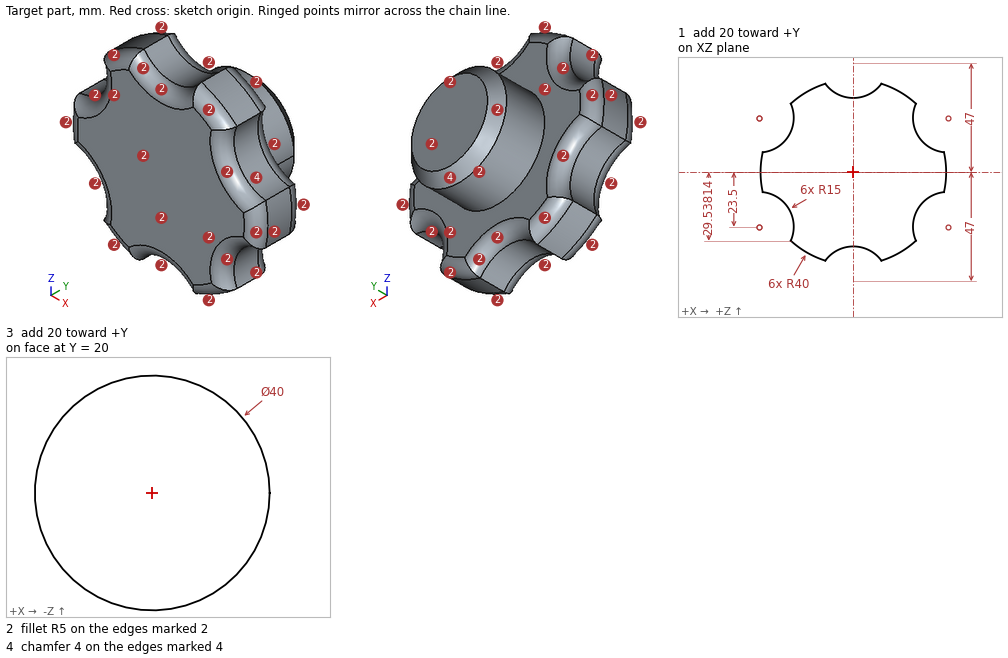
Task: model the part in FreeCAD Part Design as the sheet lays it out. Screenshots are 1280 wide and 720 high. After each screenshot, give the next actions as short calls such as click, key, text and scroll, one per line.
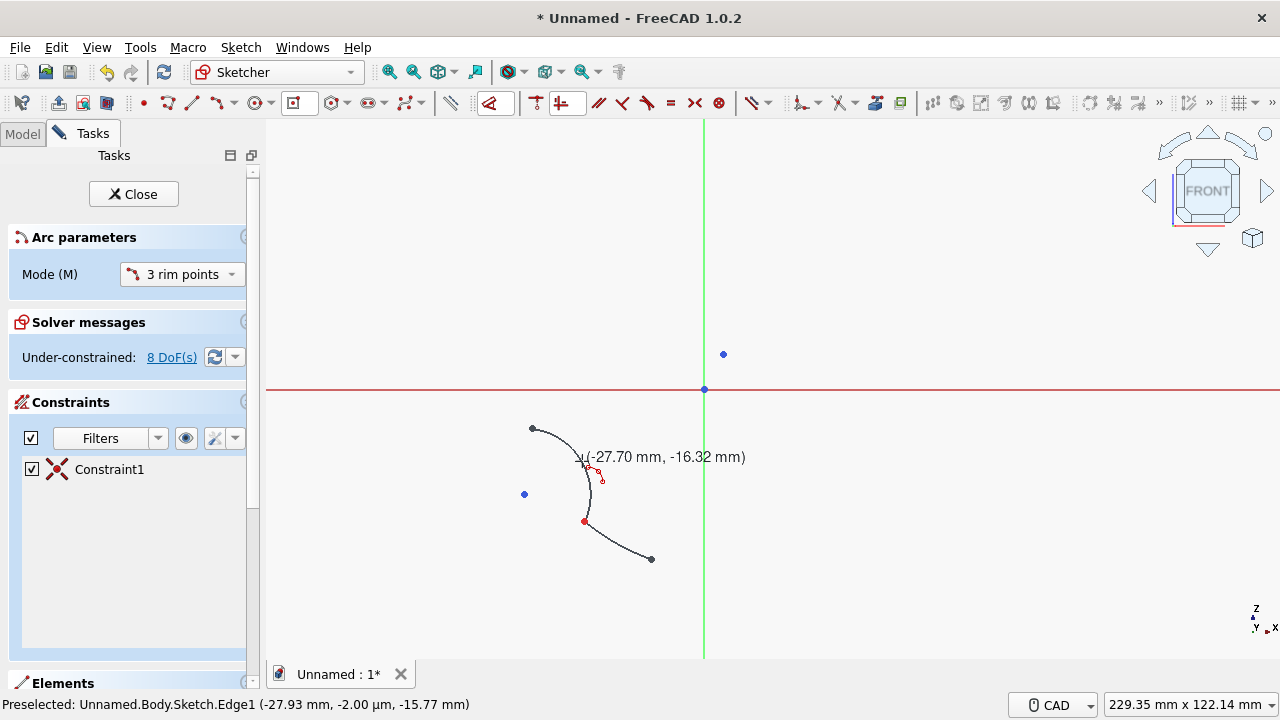
click(532, 429)
click(532, 352)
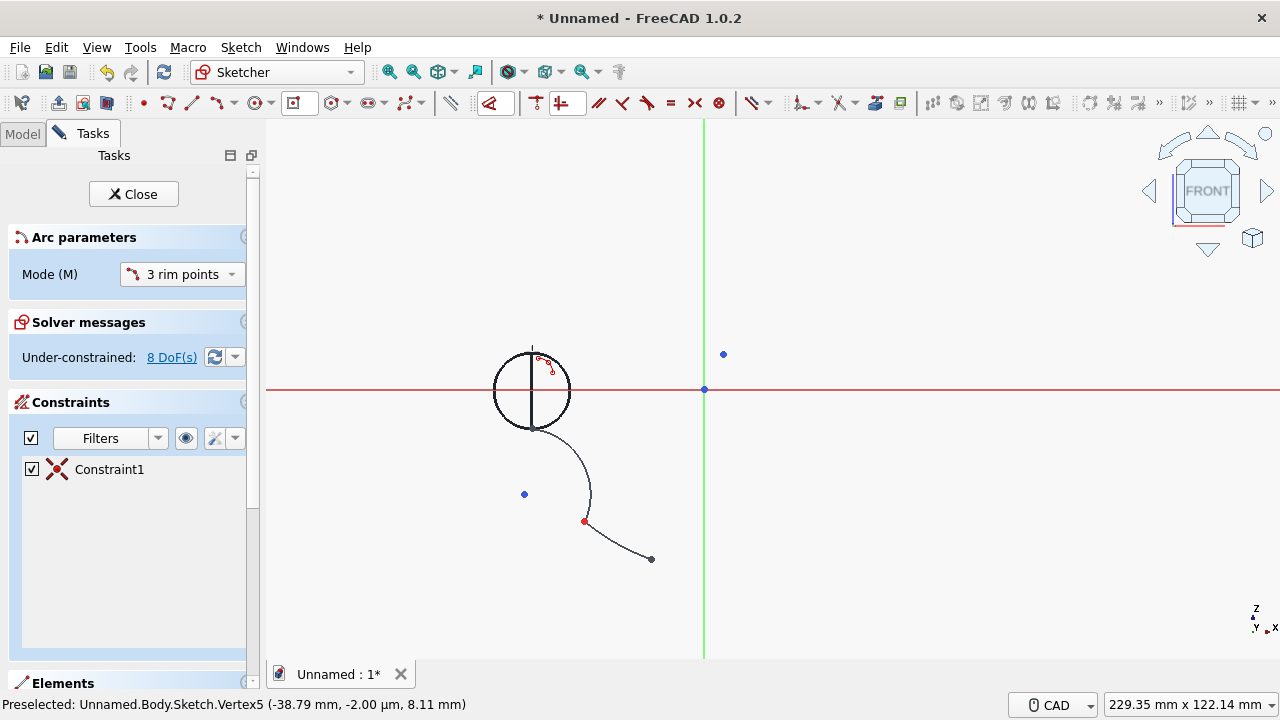
scroll(528, 382, up, 7)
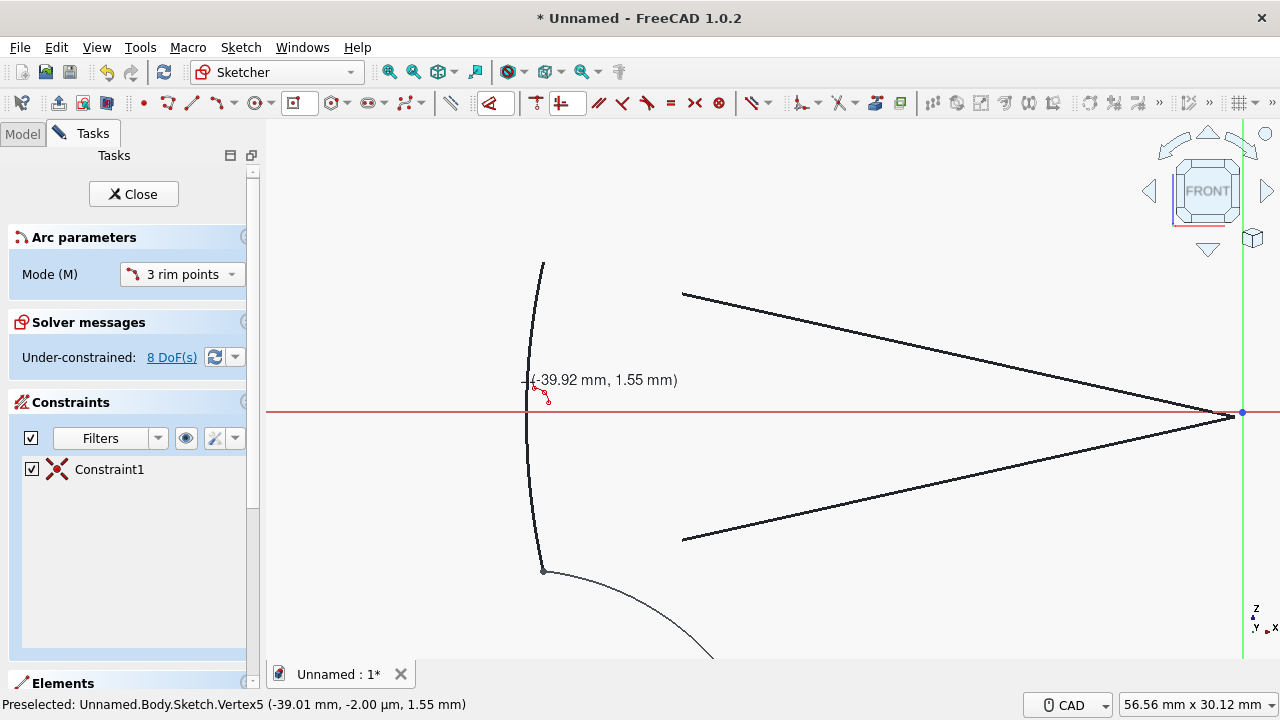
click(526, 381)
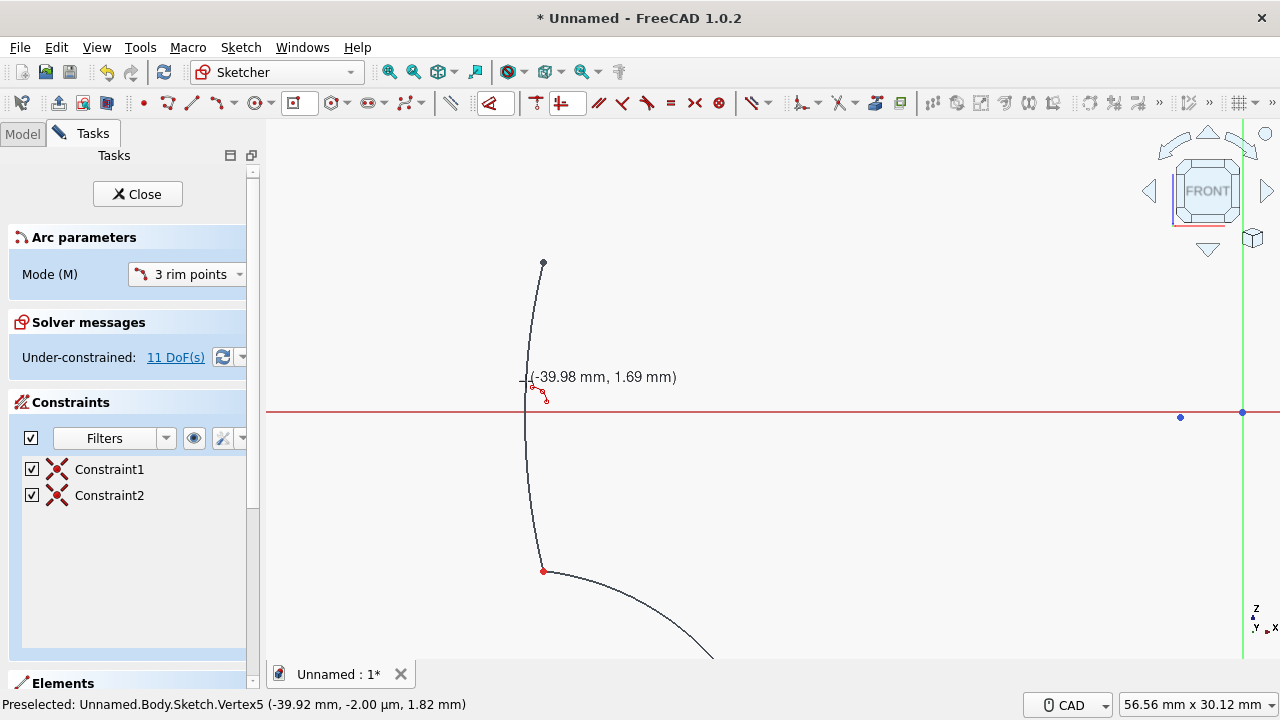
click(543, 263)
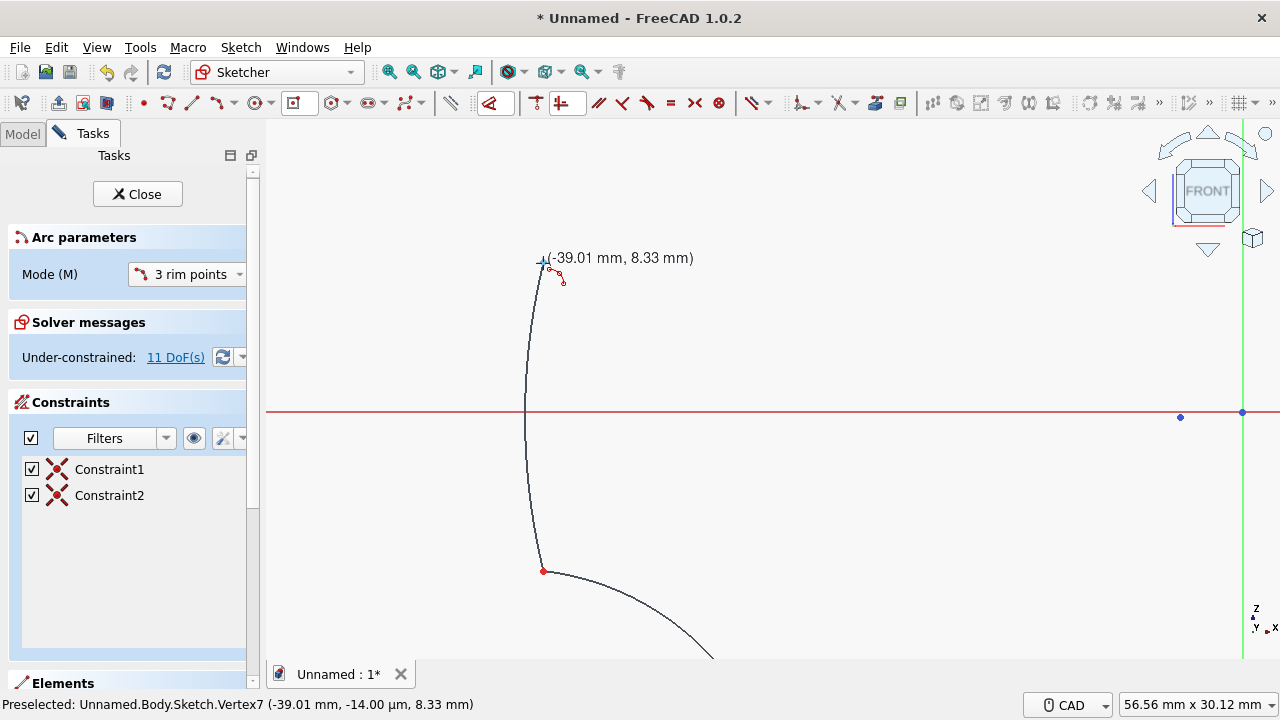
scroll(528, 381, down, 7)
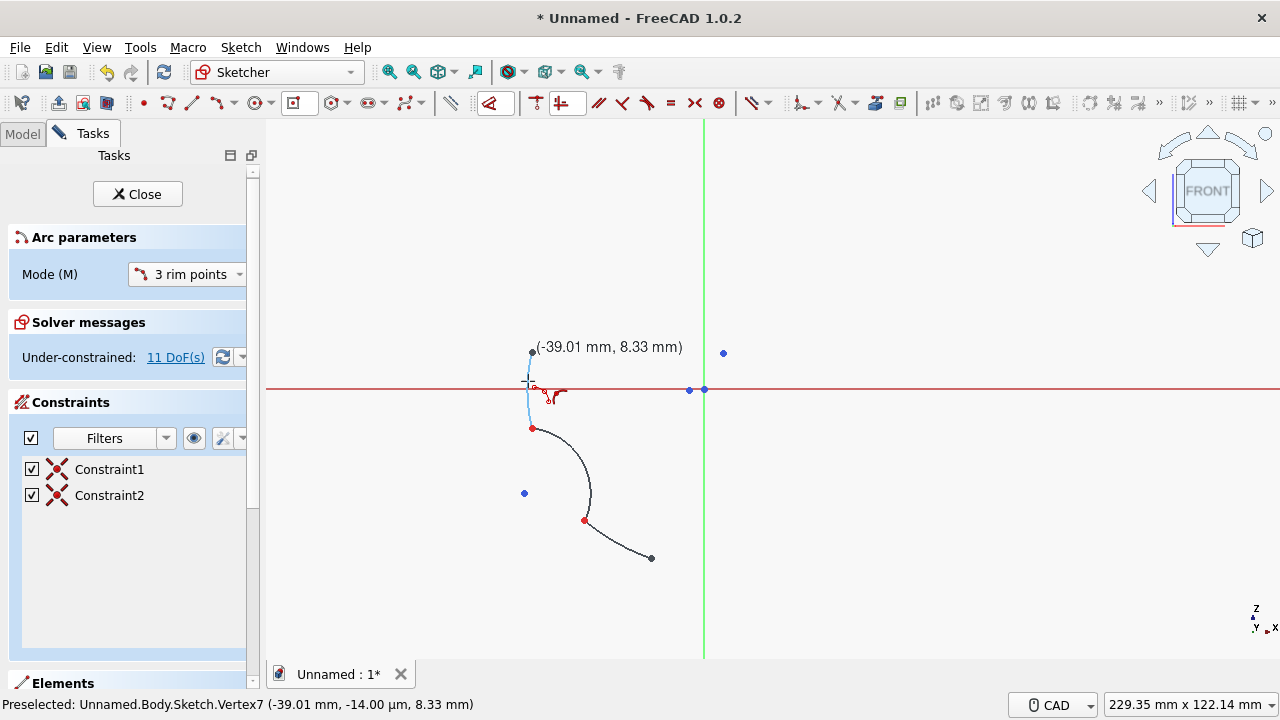
click(585, 258)
click(582, 318)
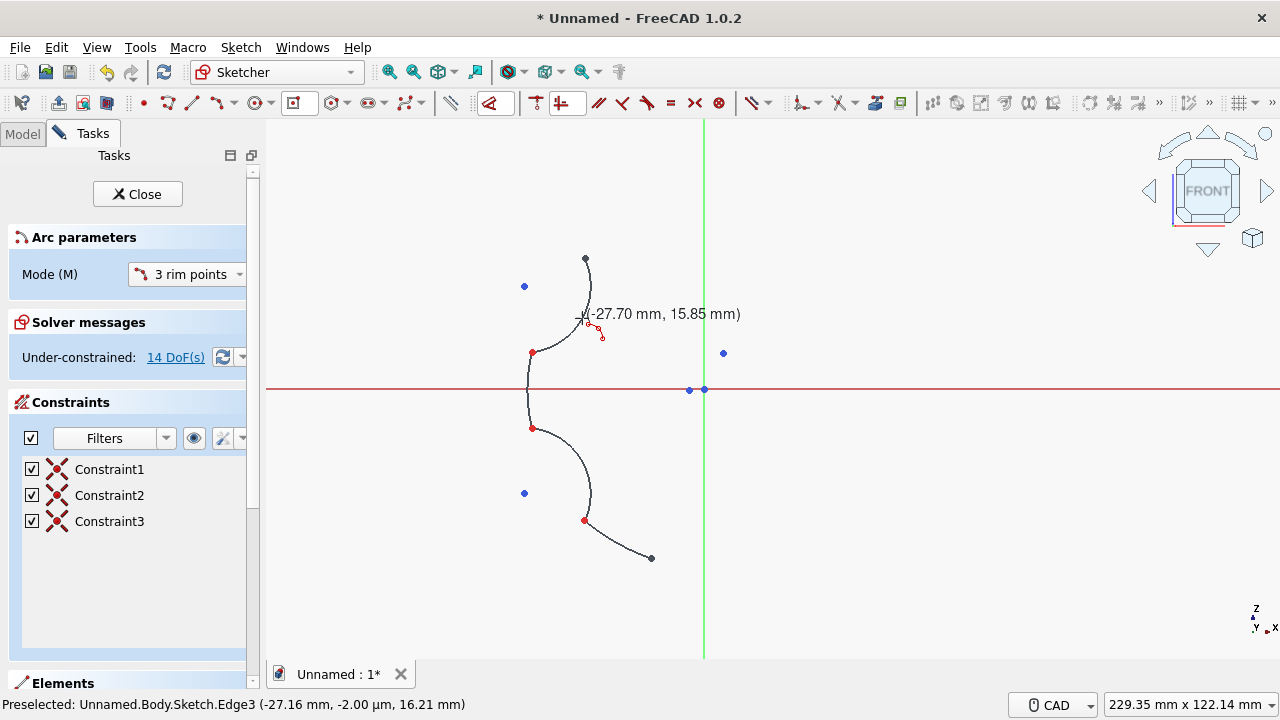
click(585, 259)
click(651, 221)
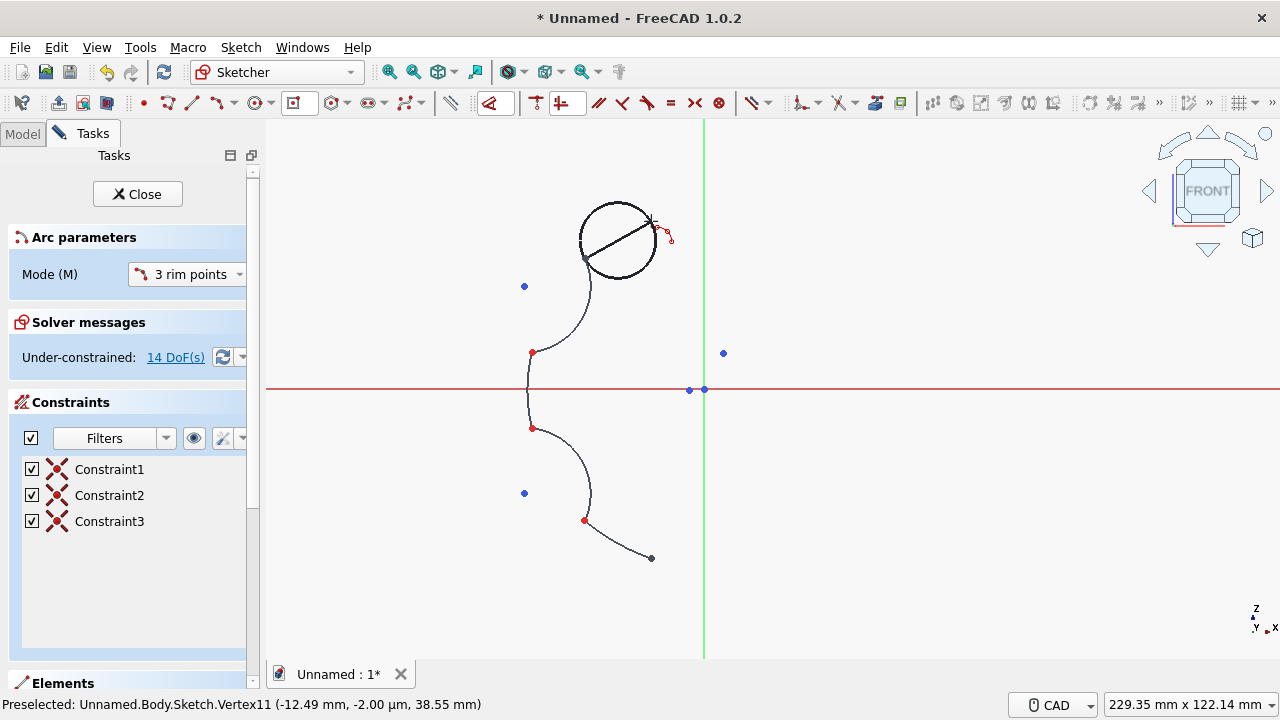
scroll(616, 236, up, 7)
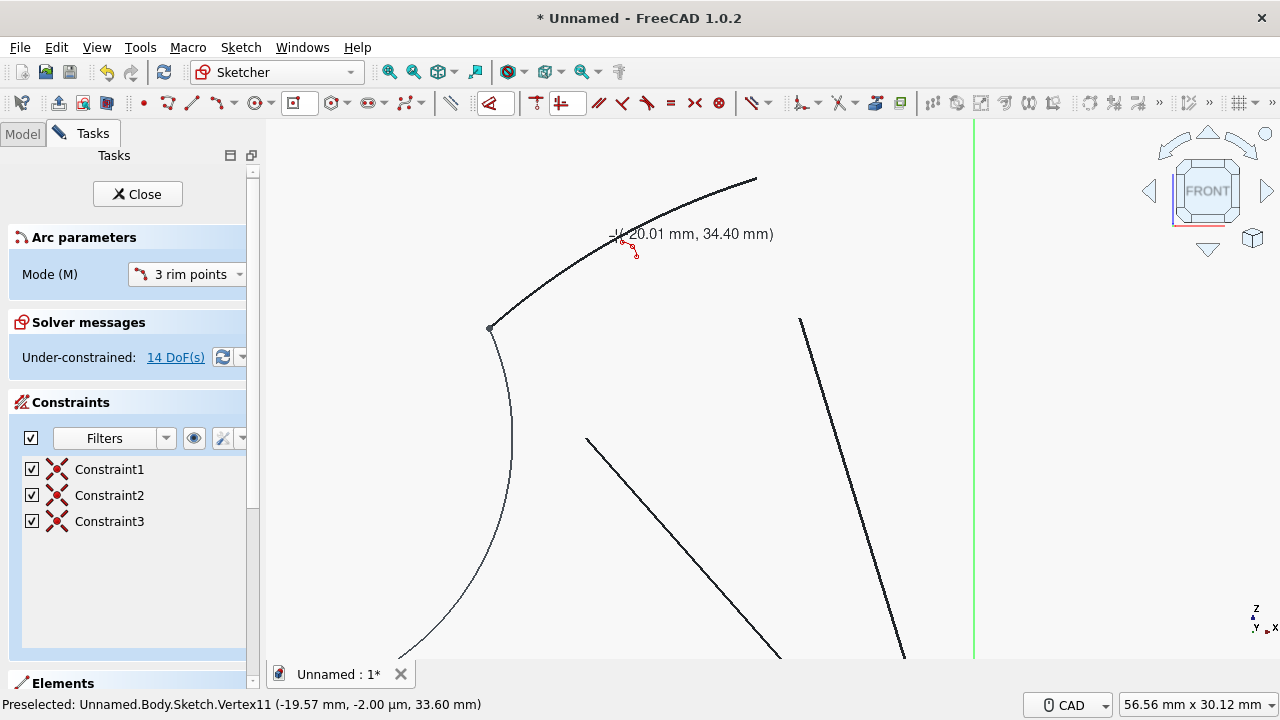
click(615, 235)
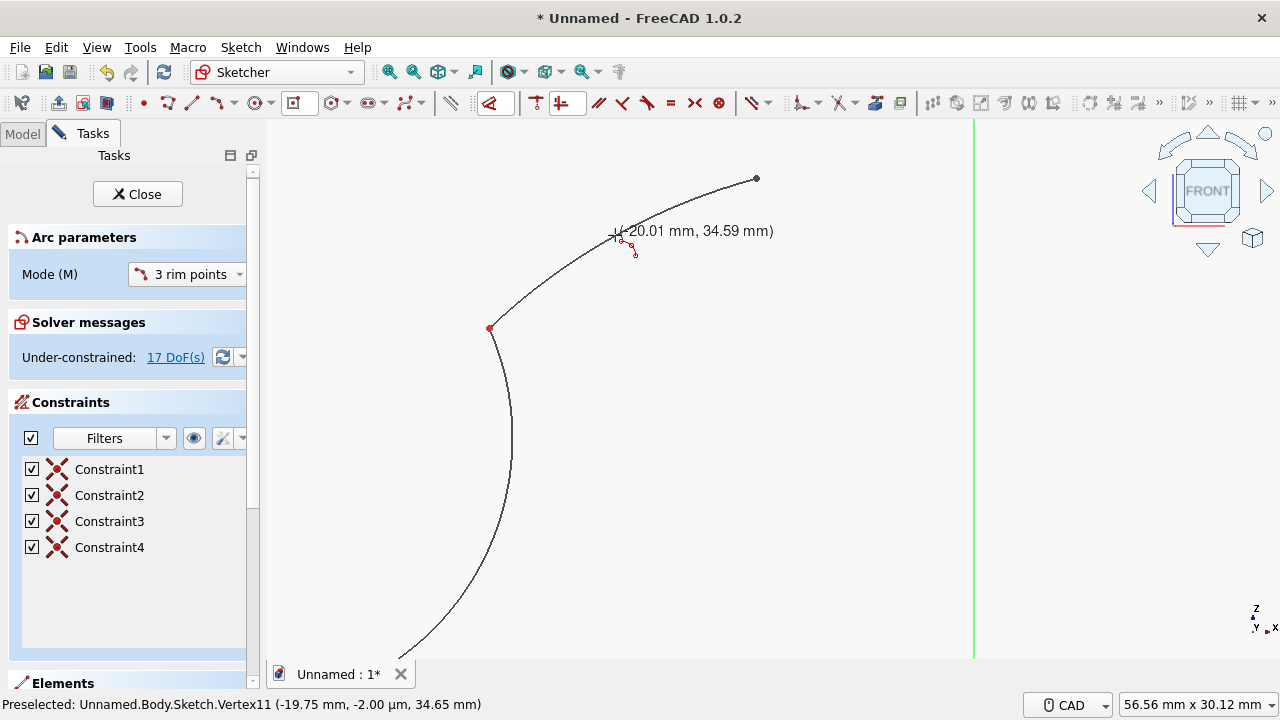
click(757, 179)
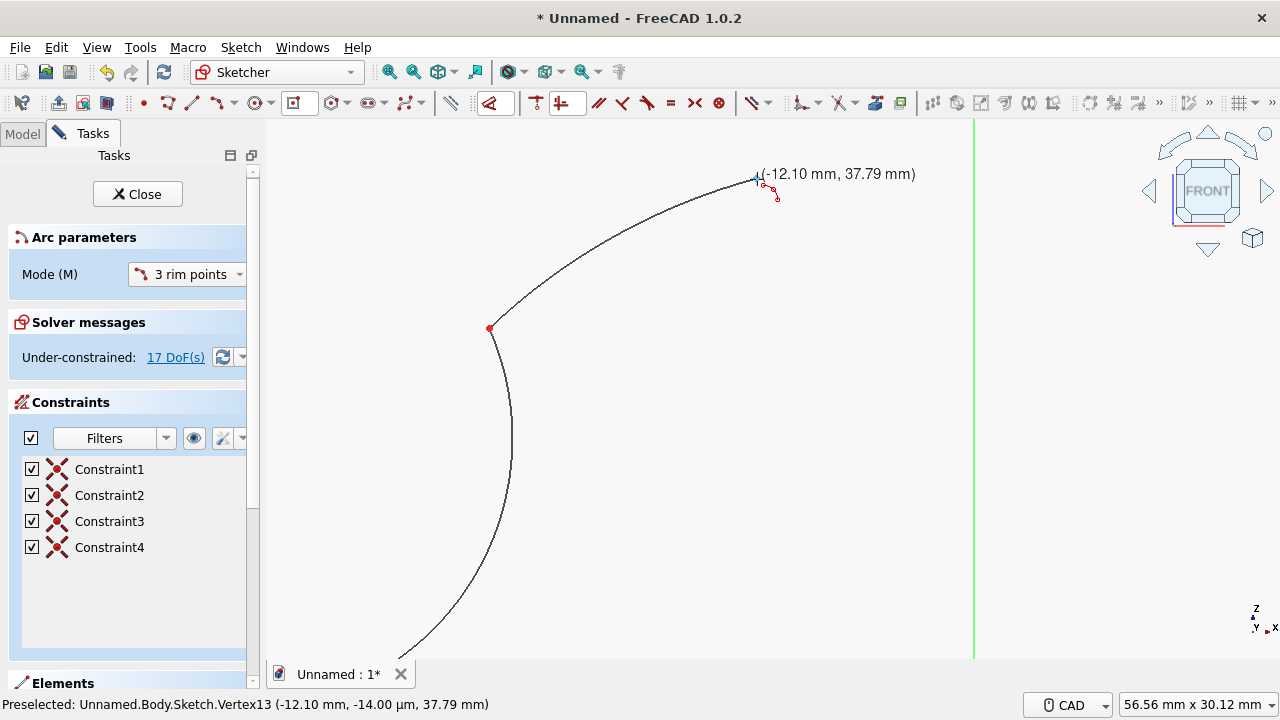
scroll(616, 236, down, 7)